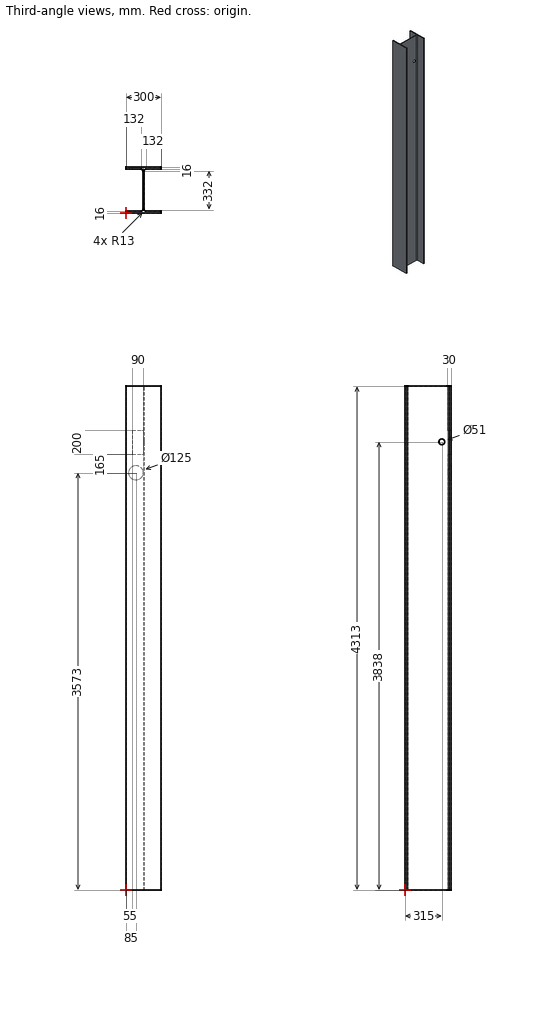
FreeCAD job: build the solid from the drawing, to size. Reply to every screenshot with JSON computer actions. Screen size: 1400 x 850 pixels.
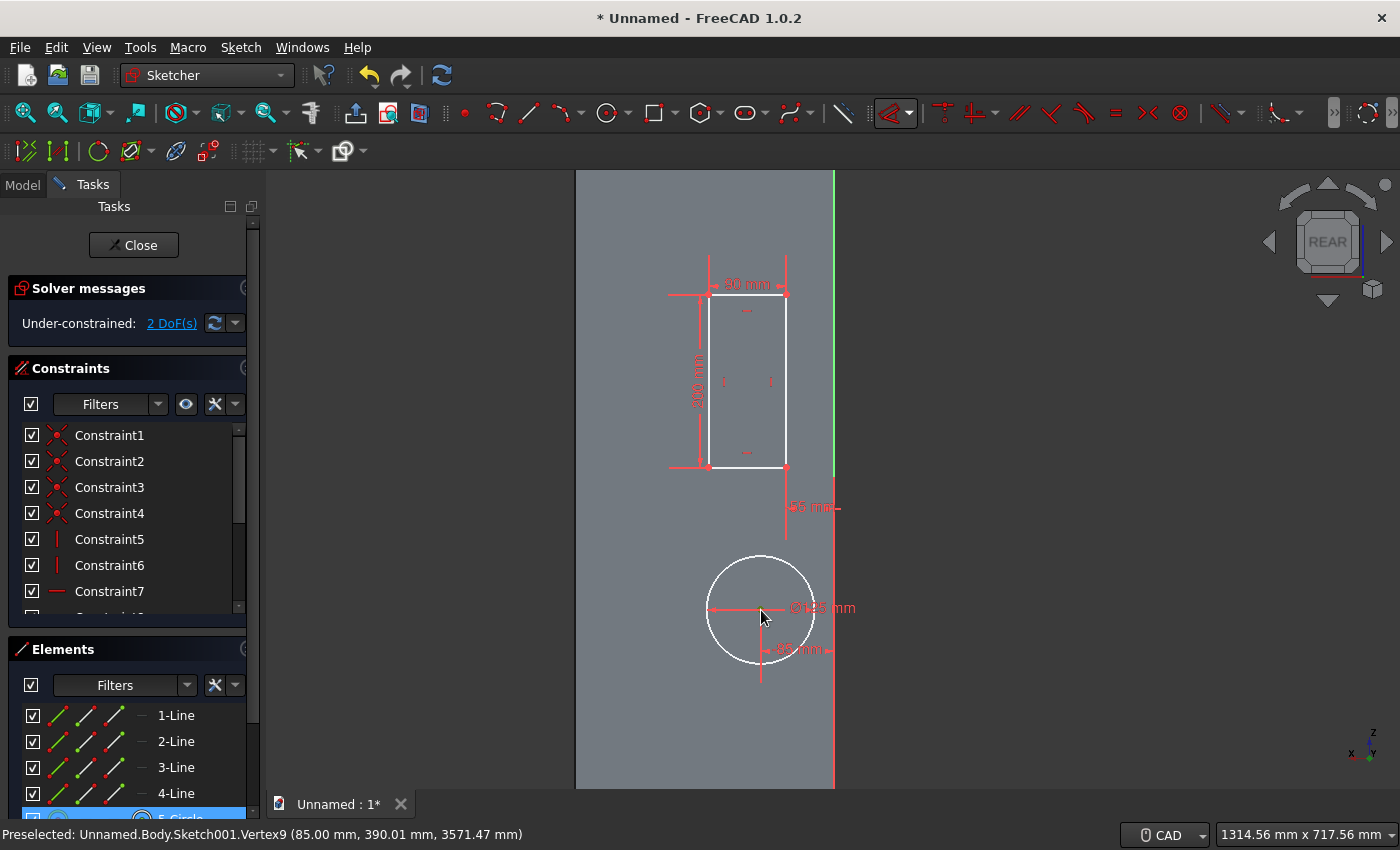
{"action": "key", "text": "i"}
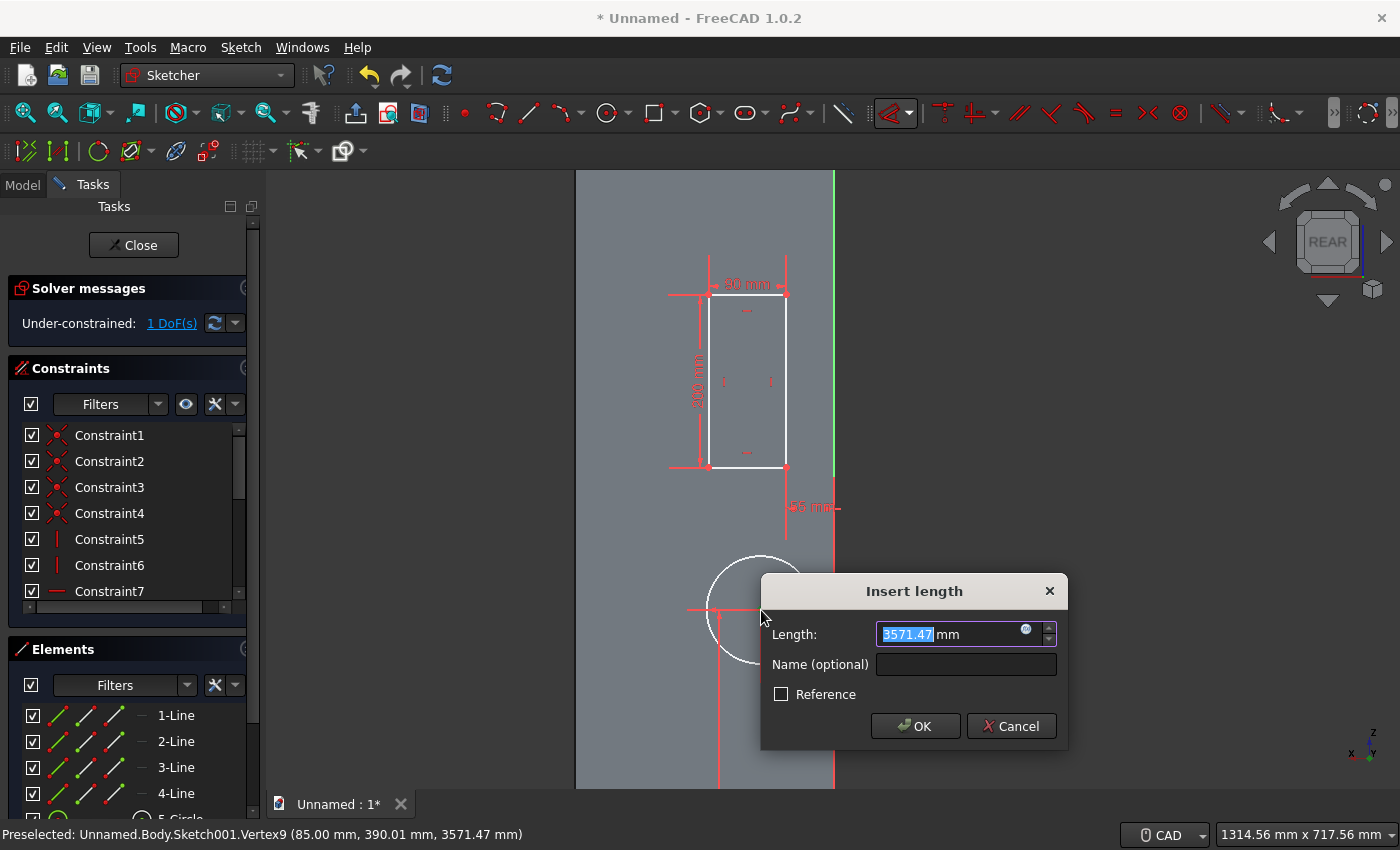
{"action": "type", "text": "3573"}
{"action": "key", "text": "Return"}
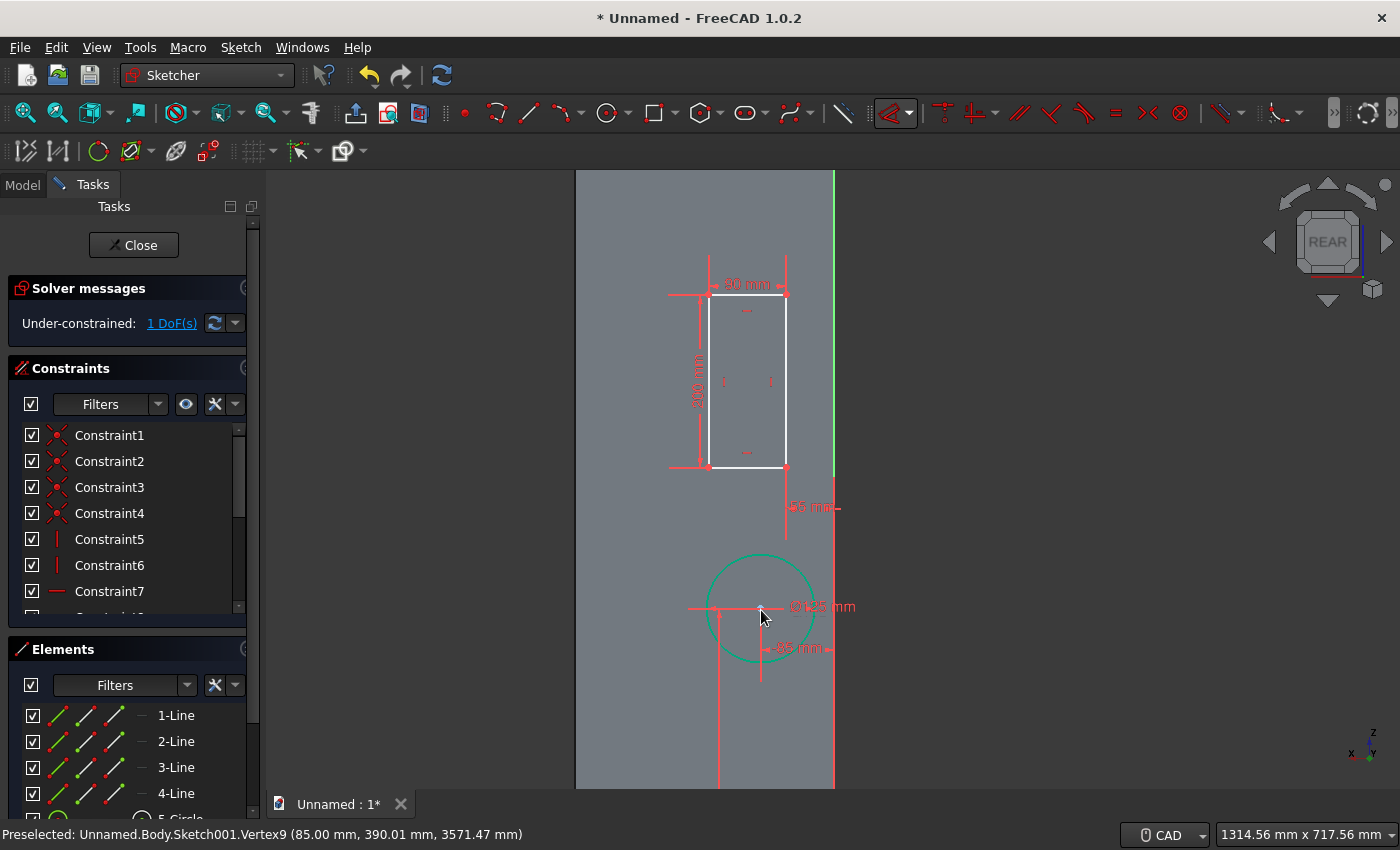
{"action": "left_click", "coordinate": [786, 468]}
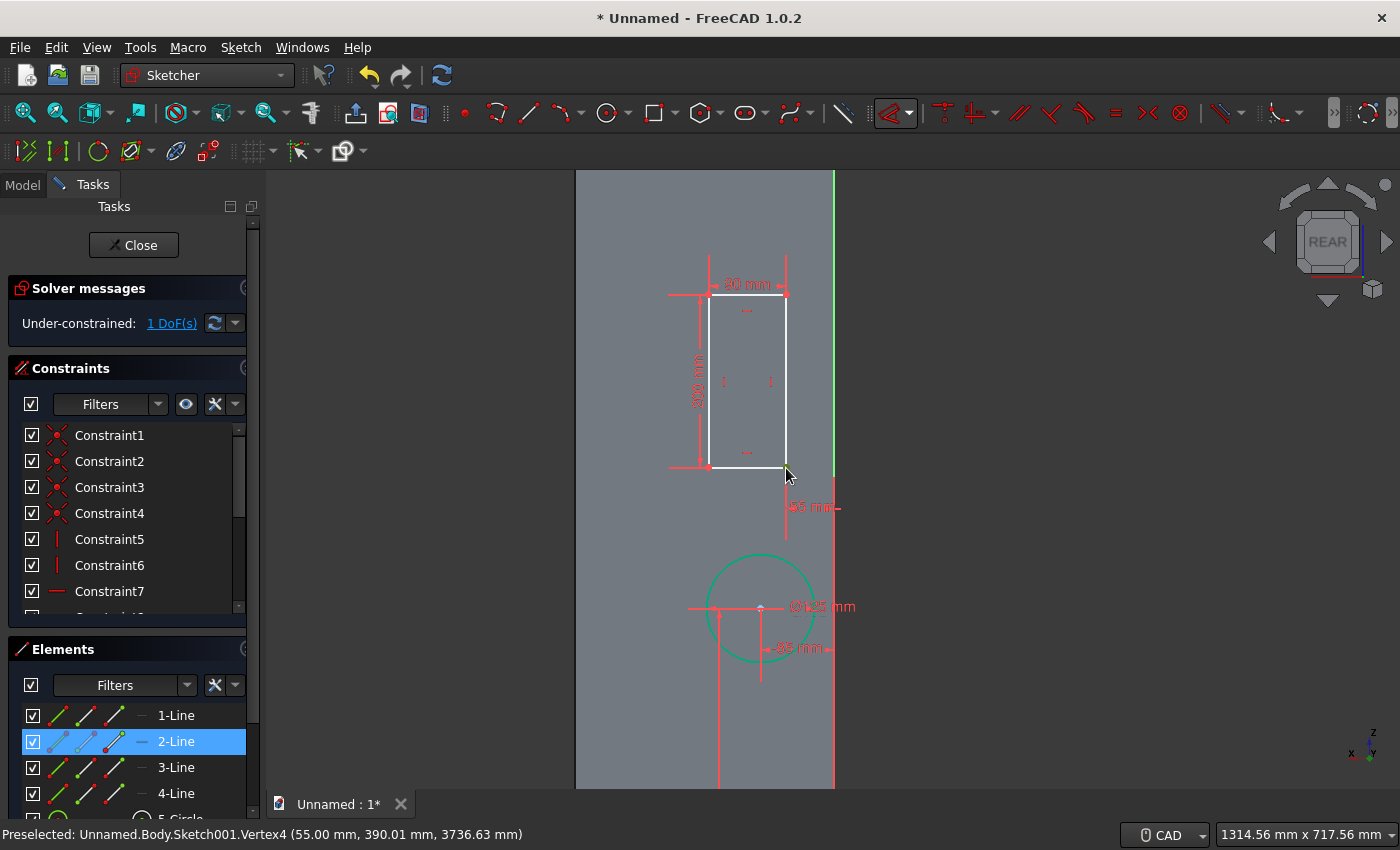
{"action": "left_click", "coordinate": [761, 609]}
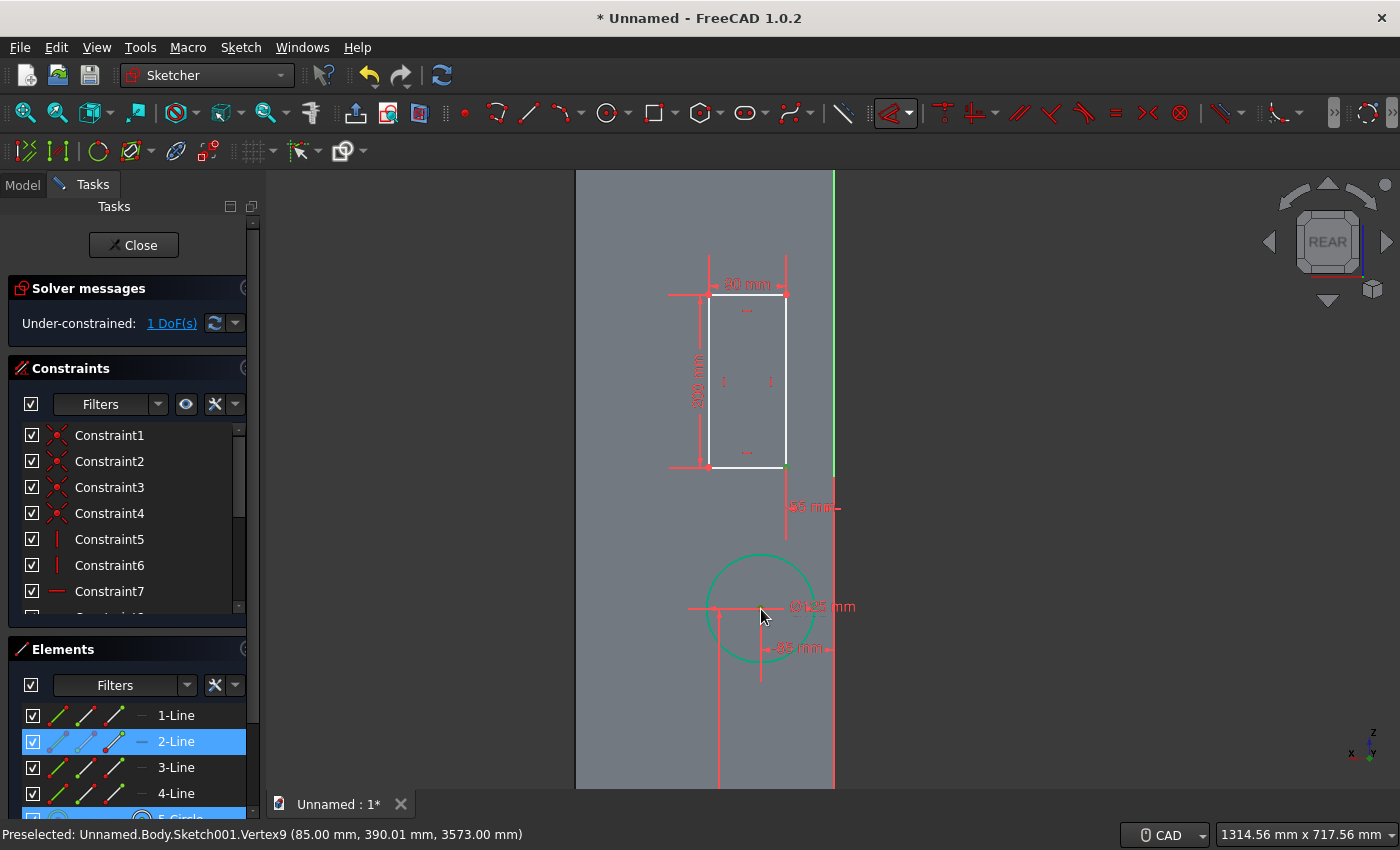
{"action": "left_click", "coordinate": [912, 114]}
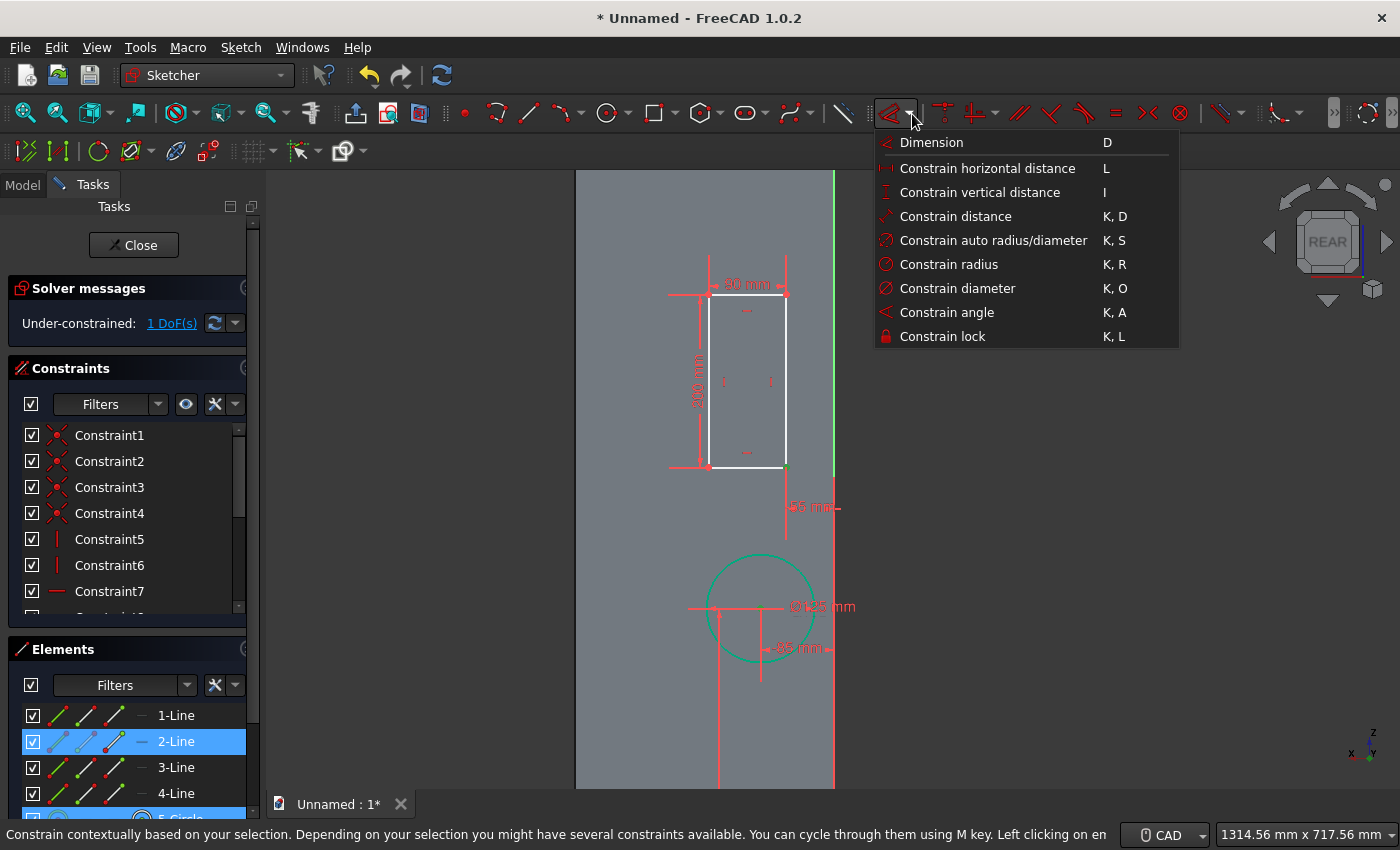
{"action": "left_click", "coordinate": [1027, 192]}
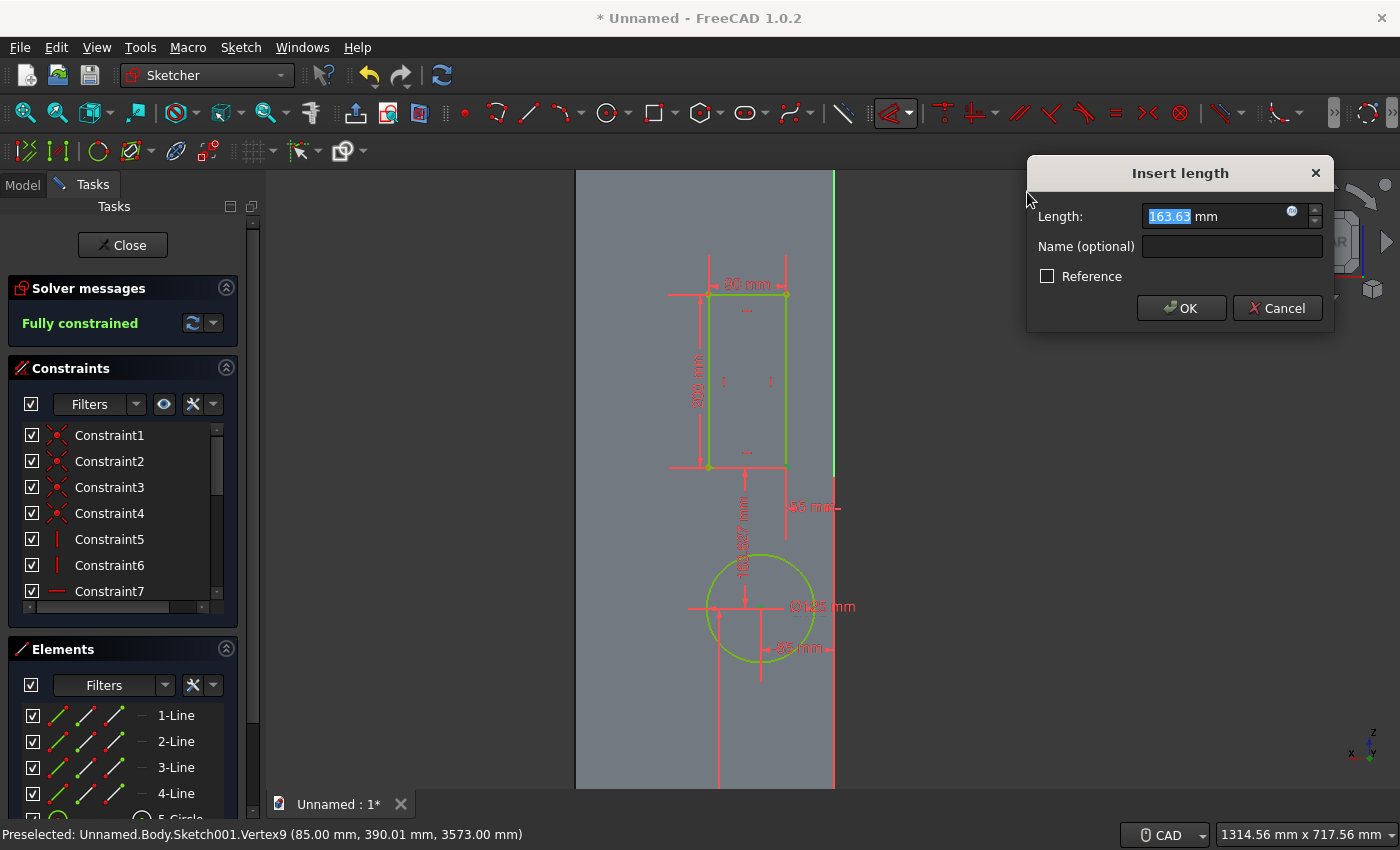
{"action": "type", "text": "165"}
{"action": "key", "text": "Return"}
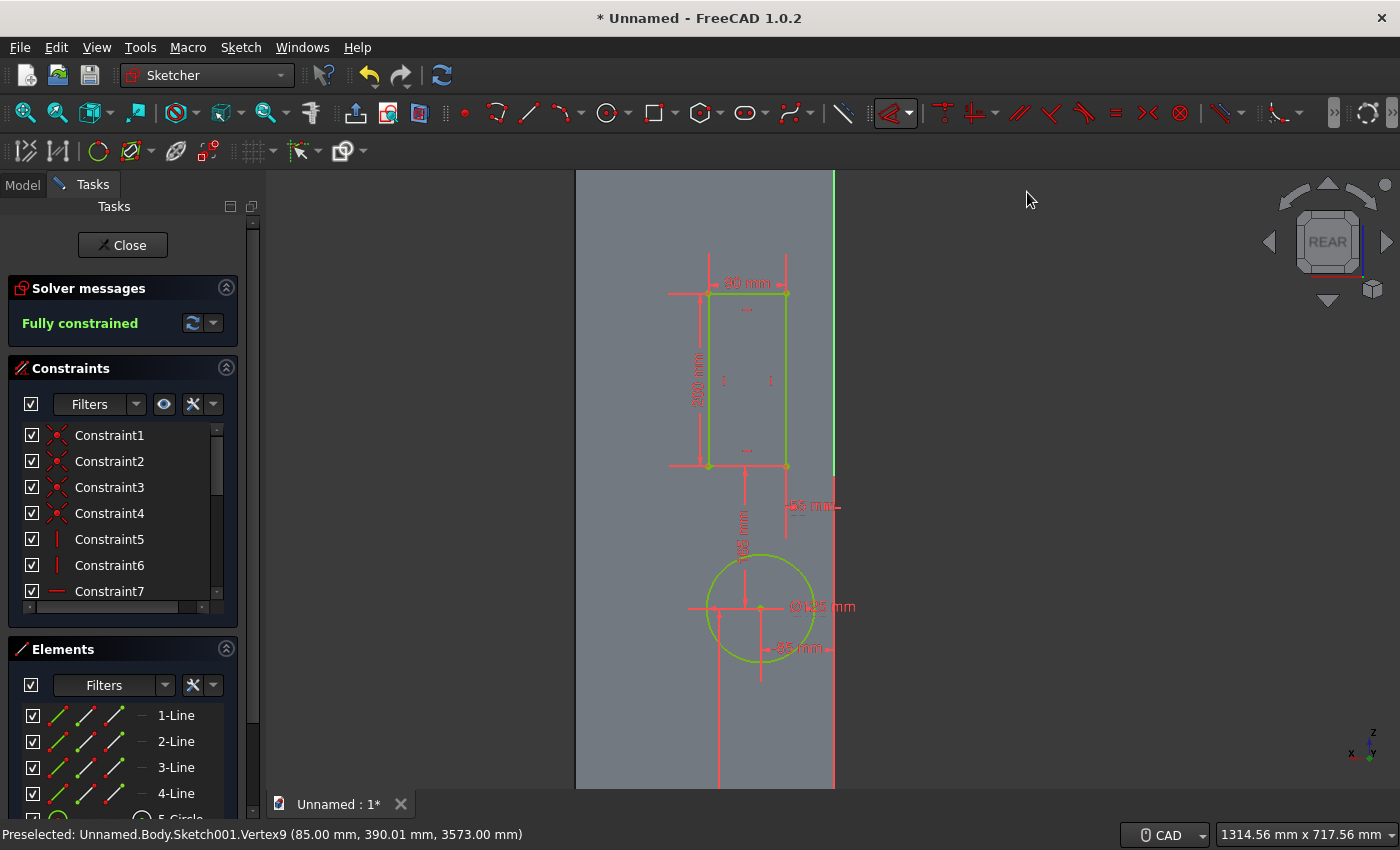
{"action": "left_click", "coordinate": [123, 245]}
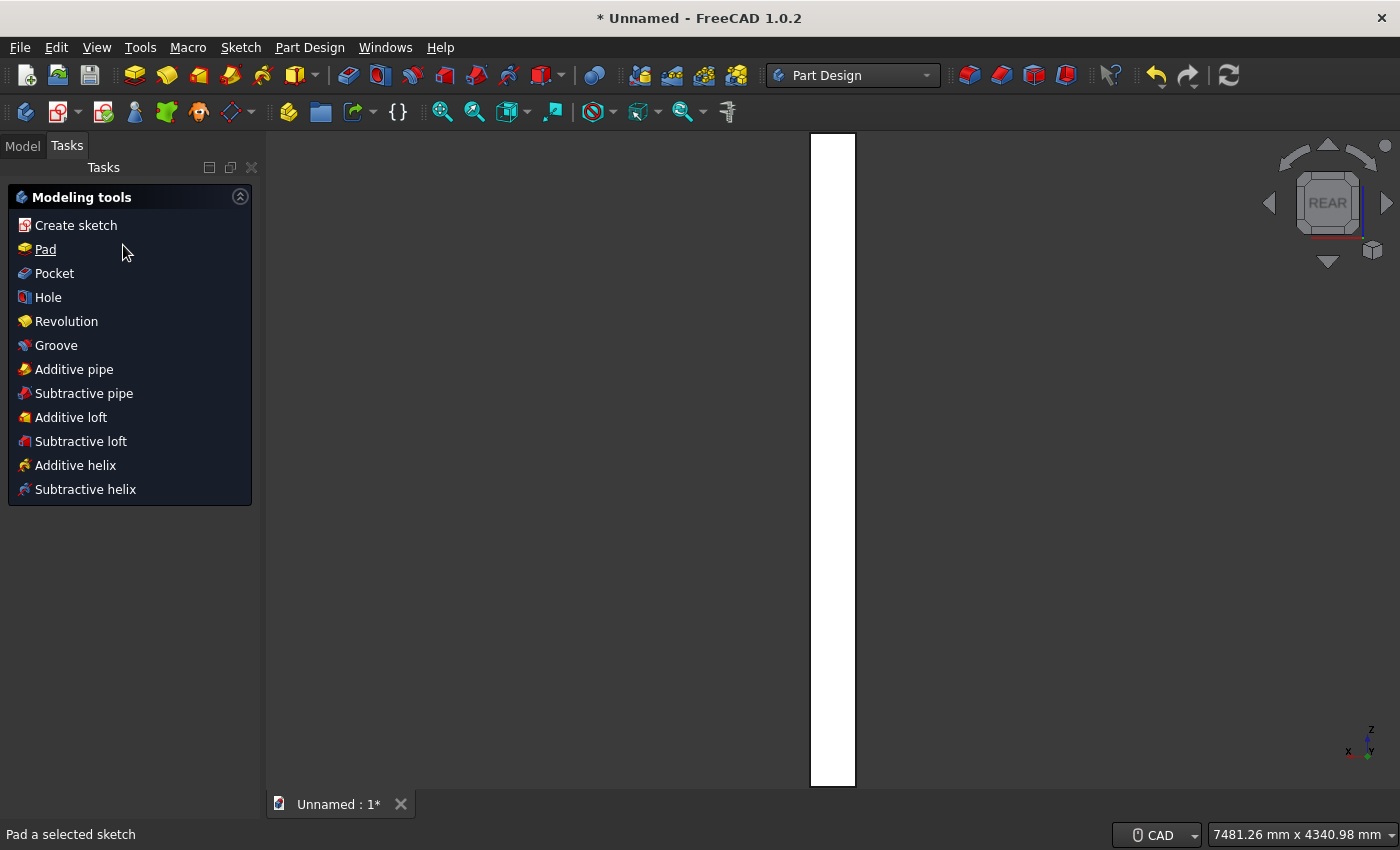
{"action": "left_click", "coordinate": [350, 76]}